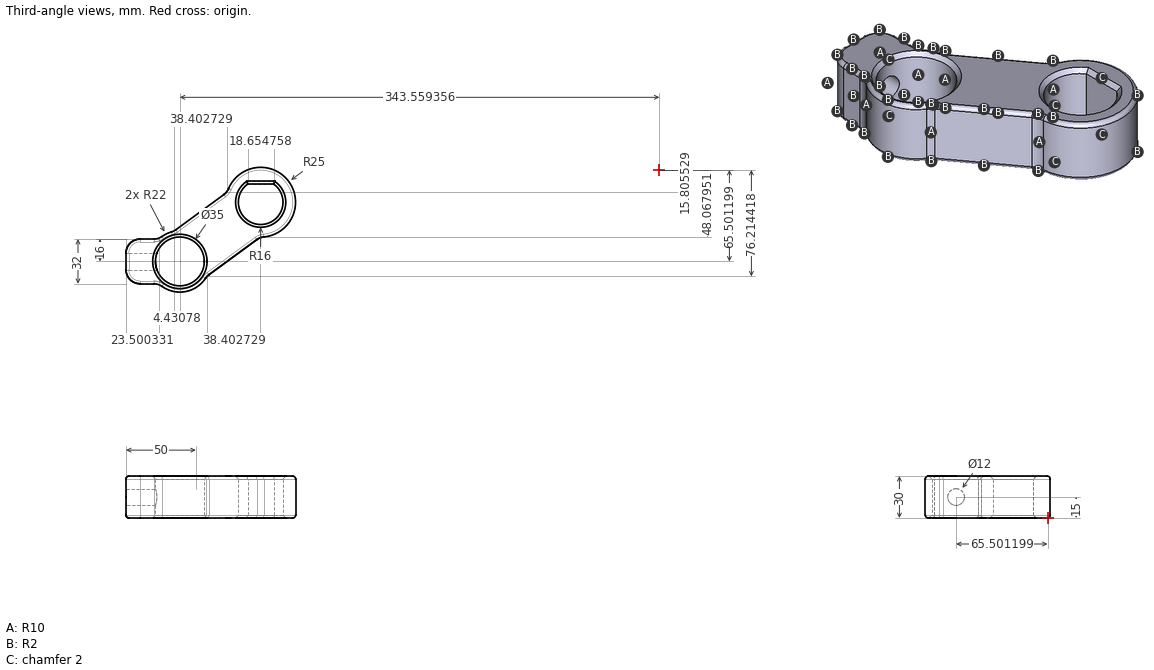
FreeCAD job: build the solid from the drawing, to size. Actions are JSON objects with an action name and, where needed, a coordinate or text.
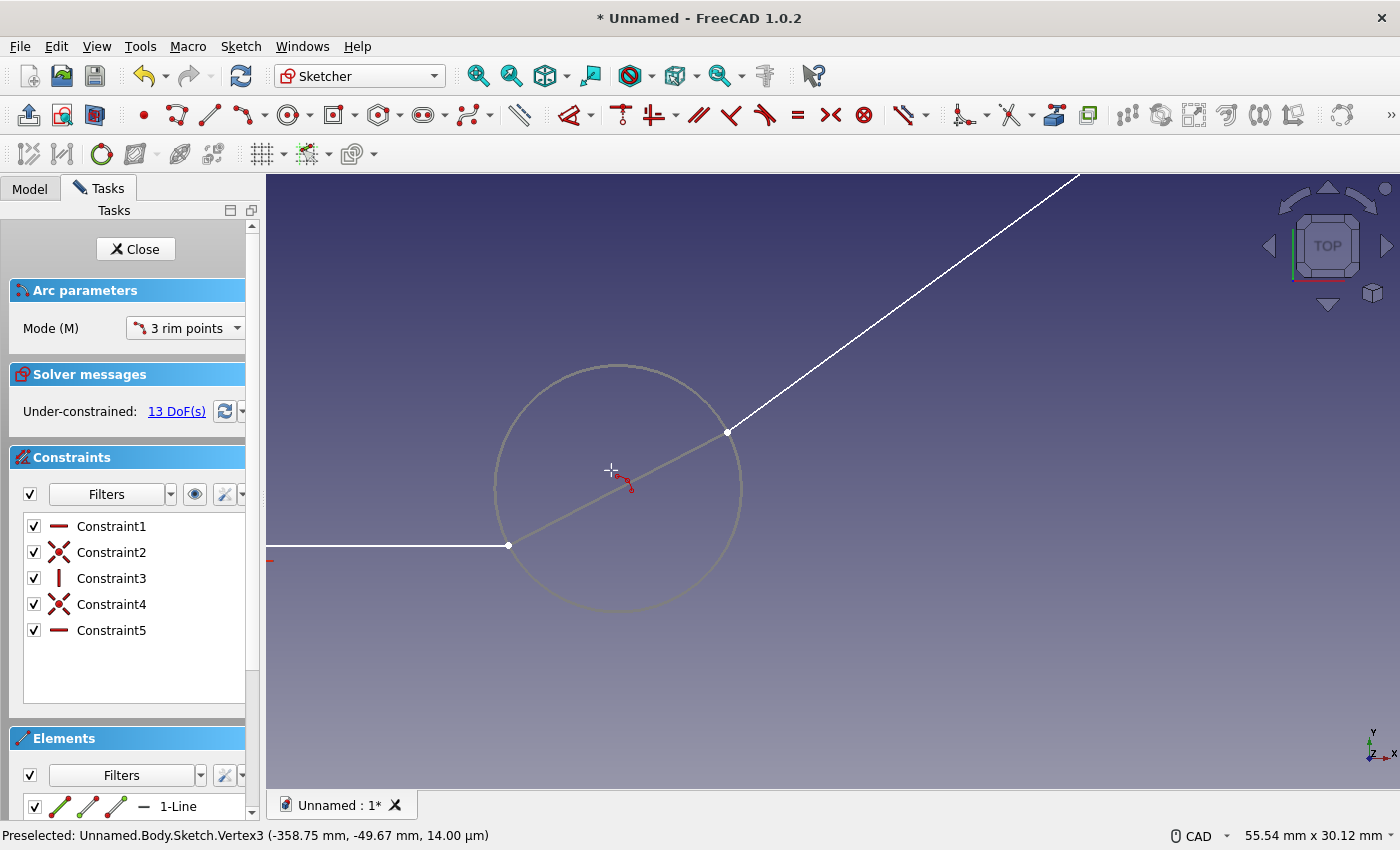
{"action": "left_click", "coordinate": [612, 470]}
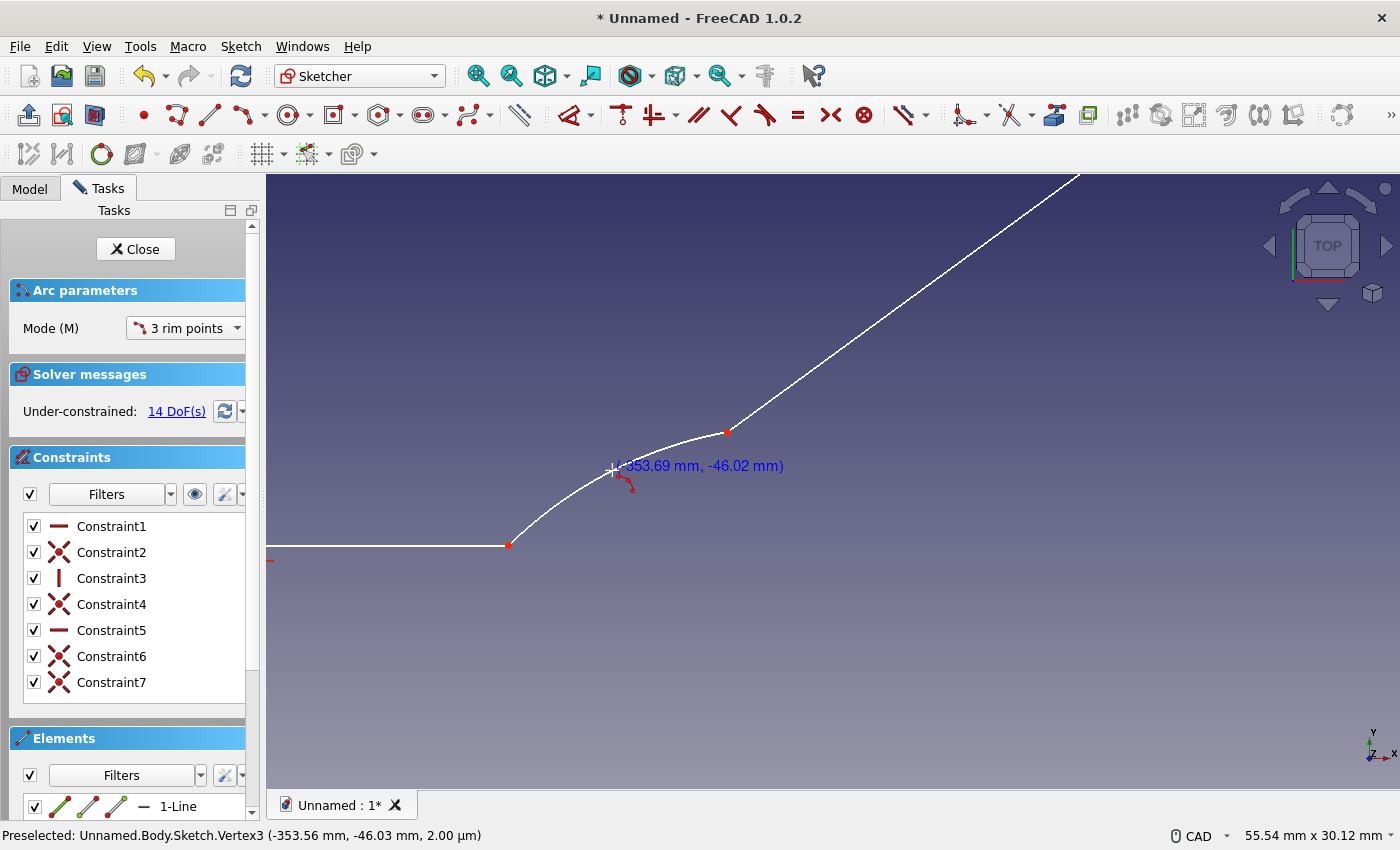
{"action": "scroll", "coordinate": [615, 473], "scroll_direction": "down", "scroll_amount": 7}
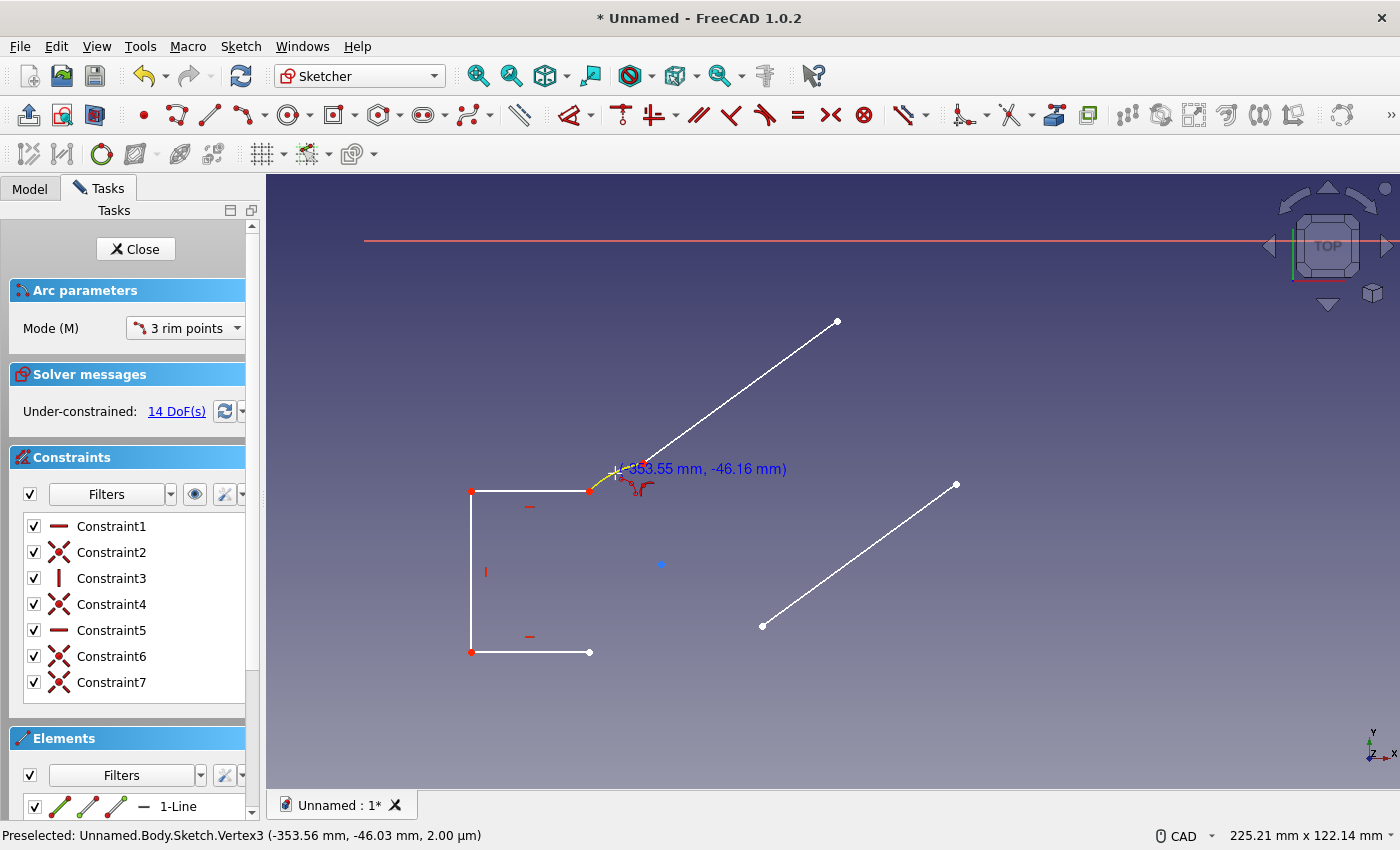
{"action": "left_click", "coordinate": [589, 652]}
{"action": "left_click", "coordinate": [762, 626]}
{"action": "left_click", "coordinate": [682, 680]}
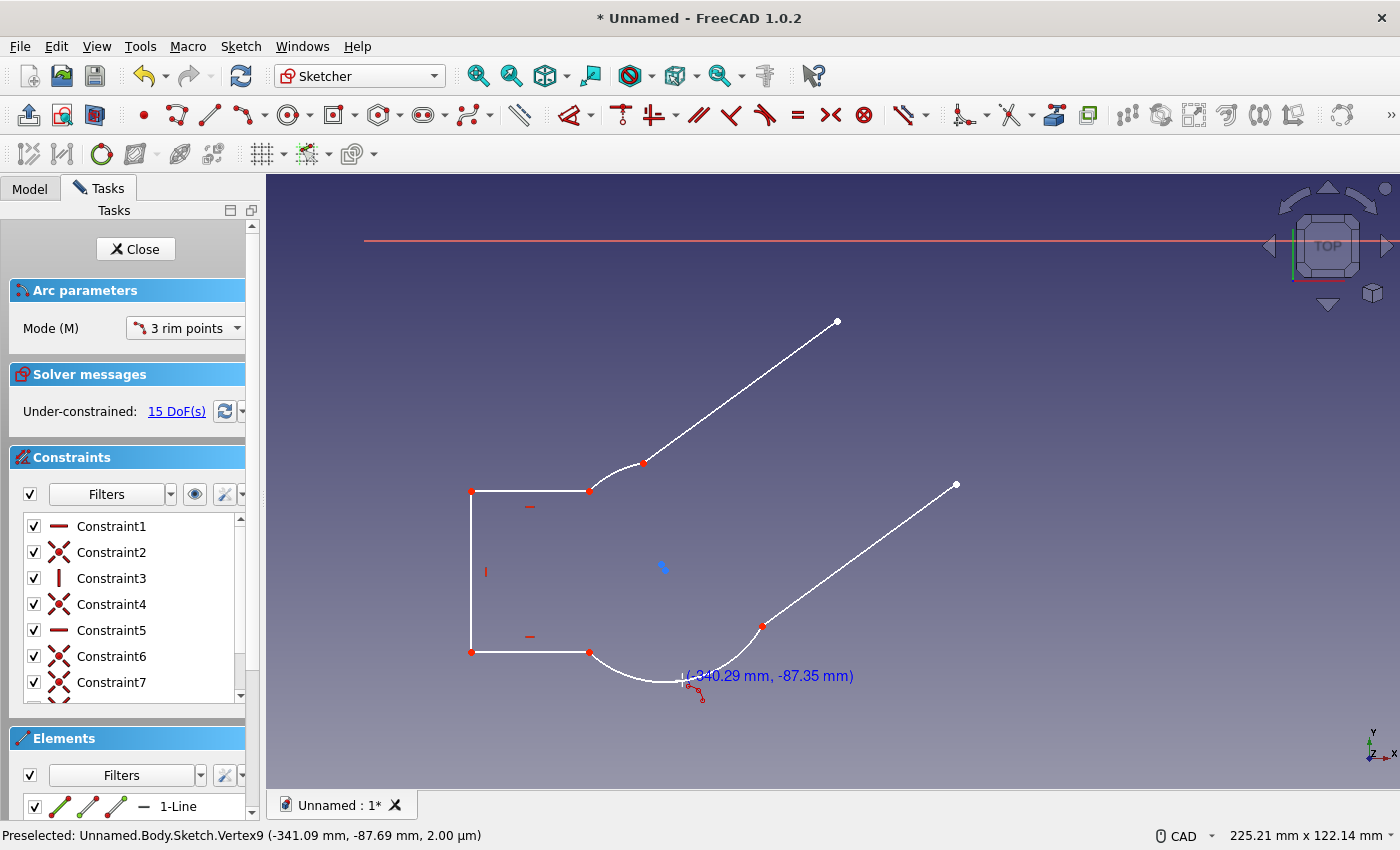
{"action": "left_click", "coordinate": [956, 484]}
{"action": "left_click", "coordinate": [837, 321]}
{"action": "left_click", "coordinate": [1059, 283]}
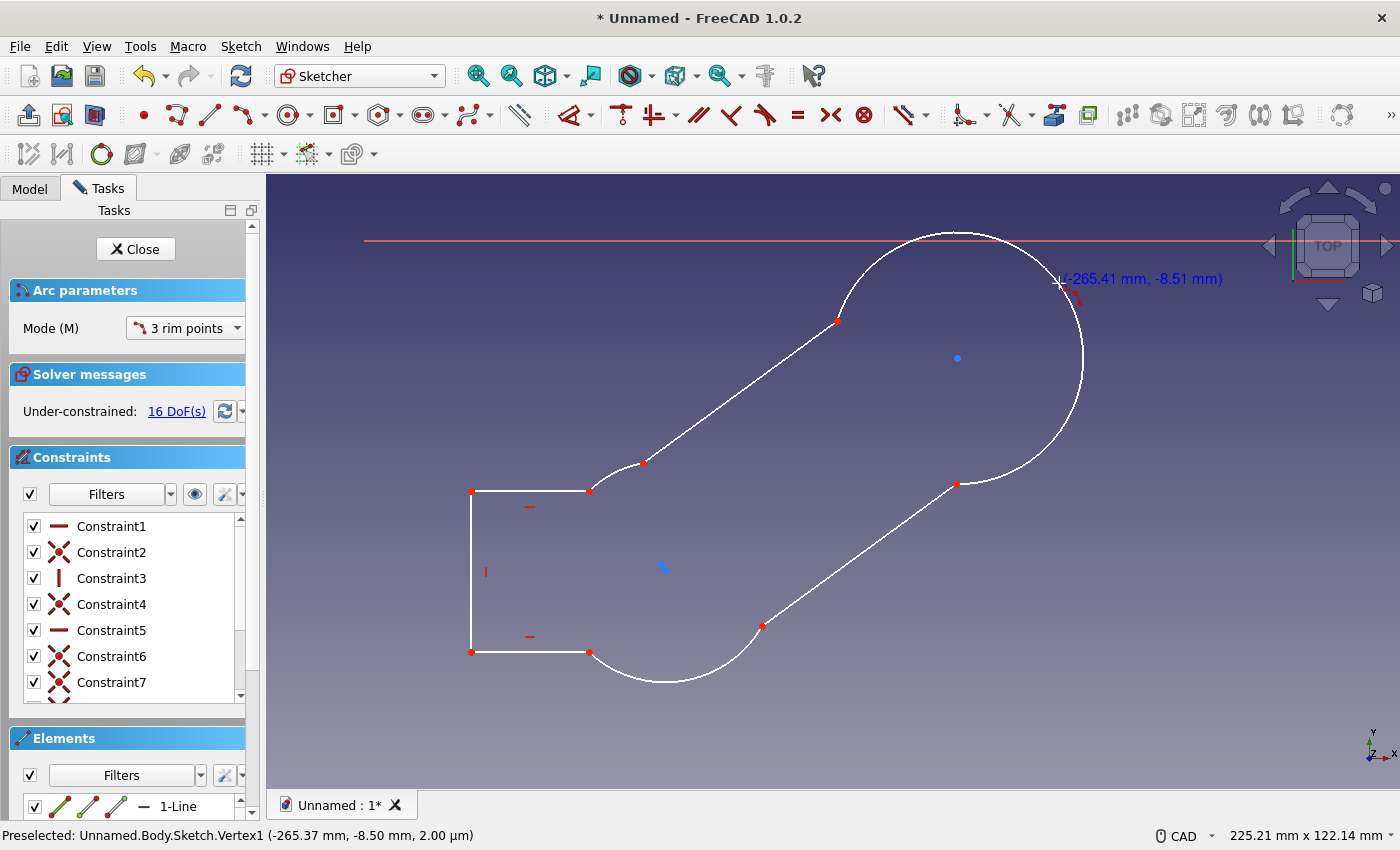
{"action": "left_click", "coordinate": [210, 116]}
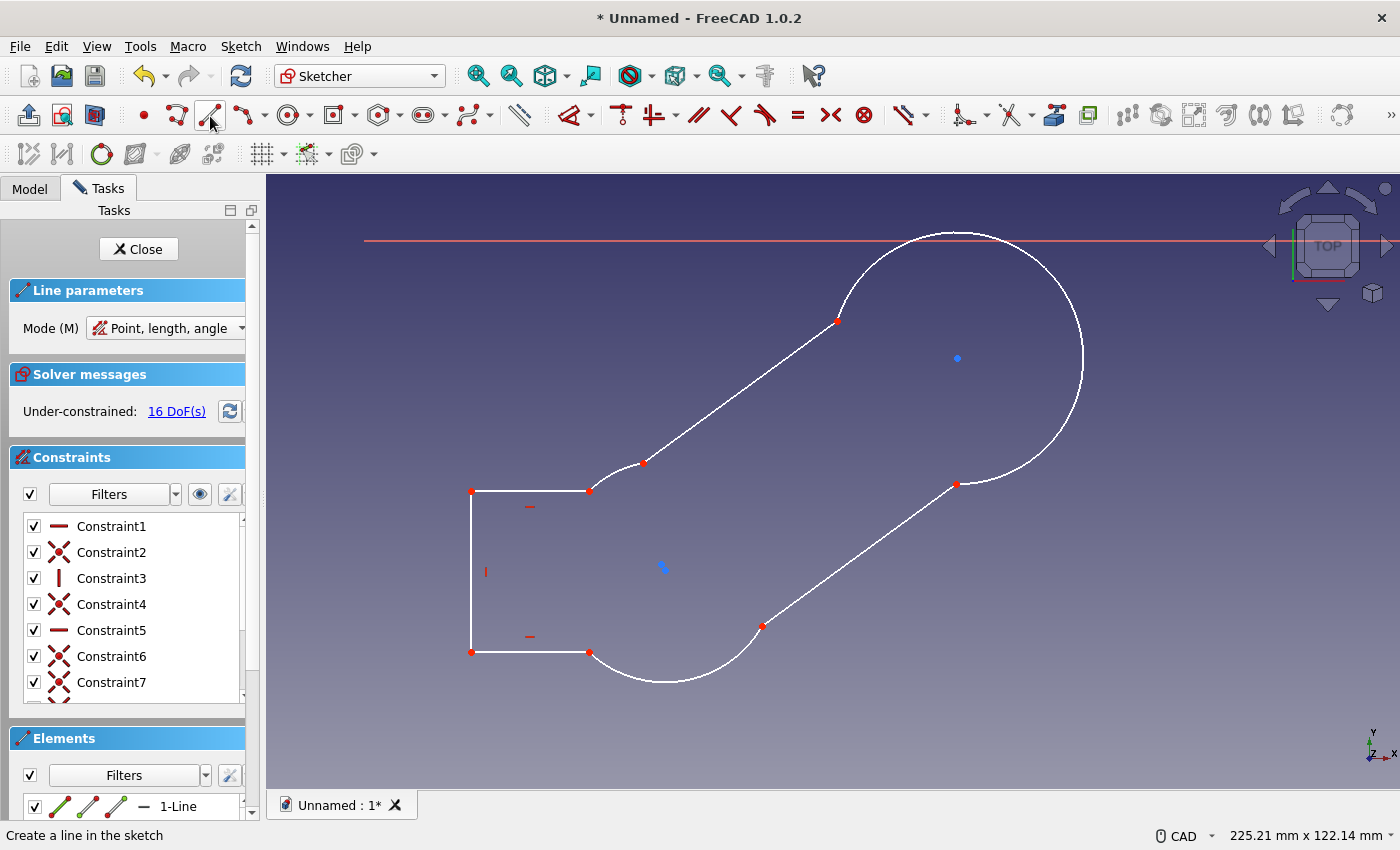
{"action": "left_click", "coordinate": [1004, 292]}
{"action": "left_click", "coordinate": [910, 292]}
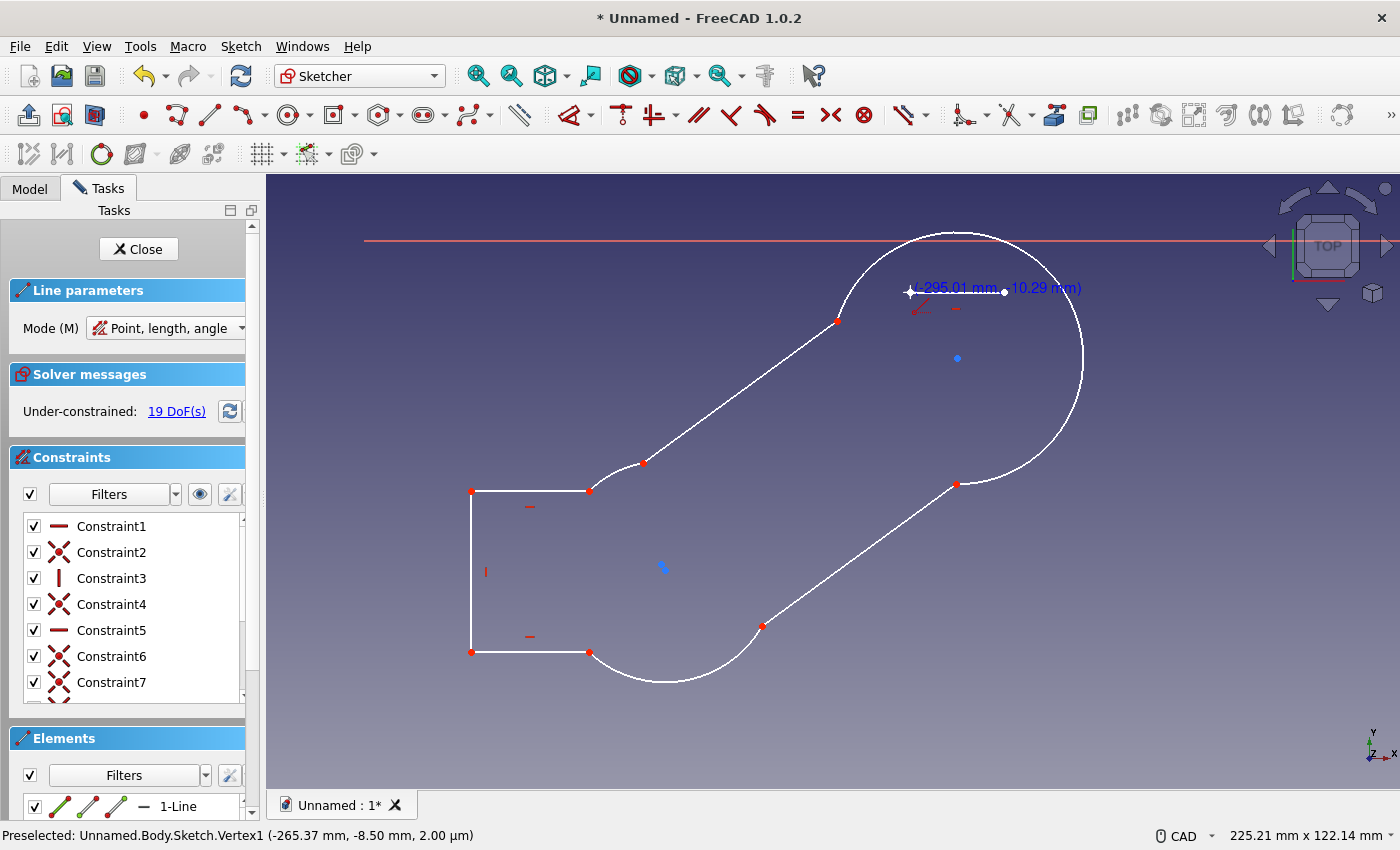
{"action": "key", "text": "g 3 a"}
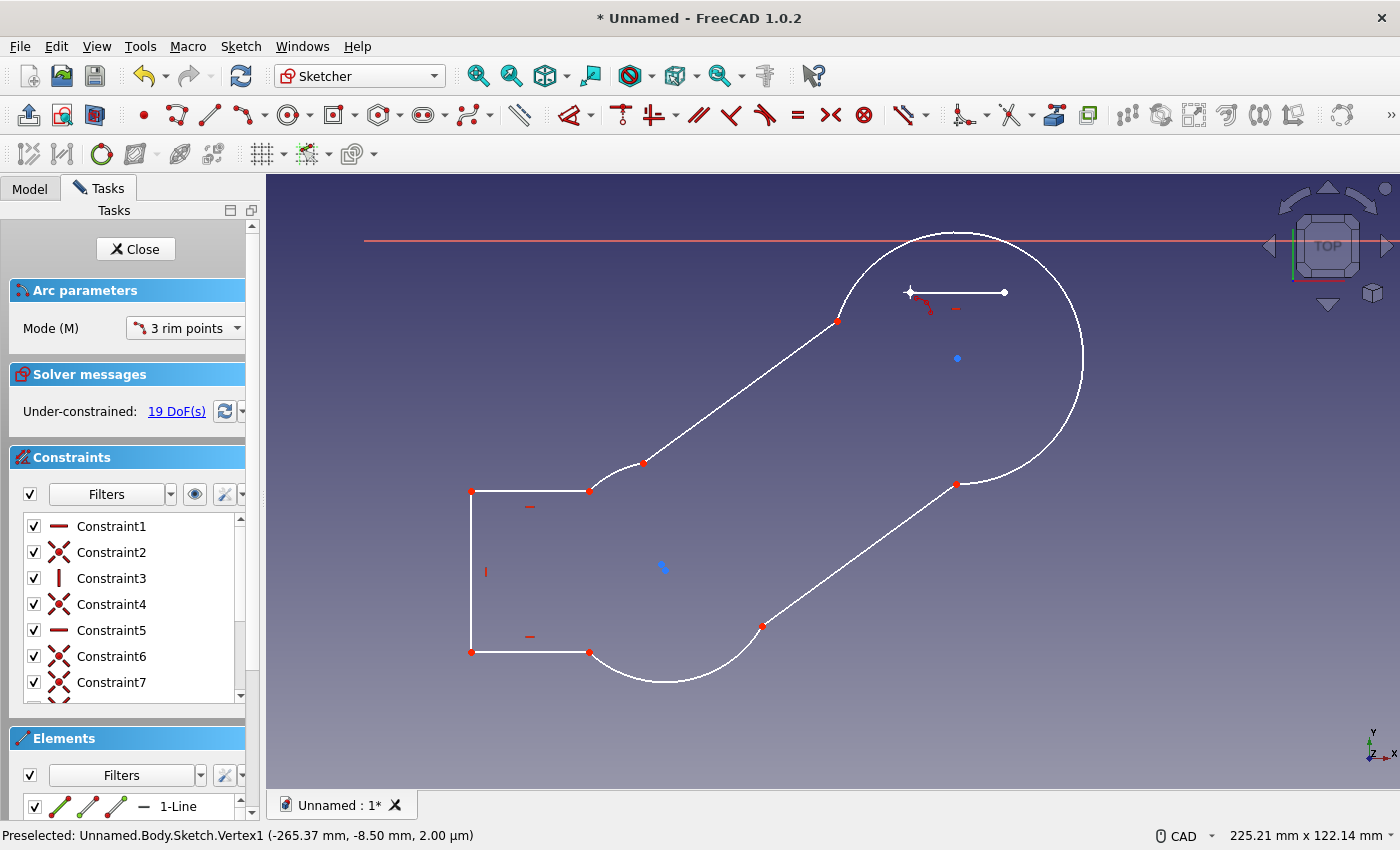
{"action": "left_click", "coordinate": [910, 293]}
{"action": "left_click", "coordinate": [1004, 293]}
{"action": "left_click", "coordinate": [957, 438]}